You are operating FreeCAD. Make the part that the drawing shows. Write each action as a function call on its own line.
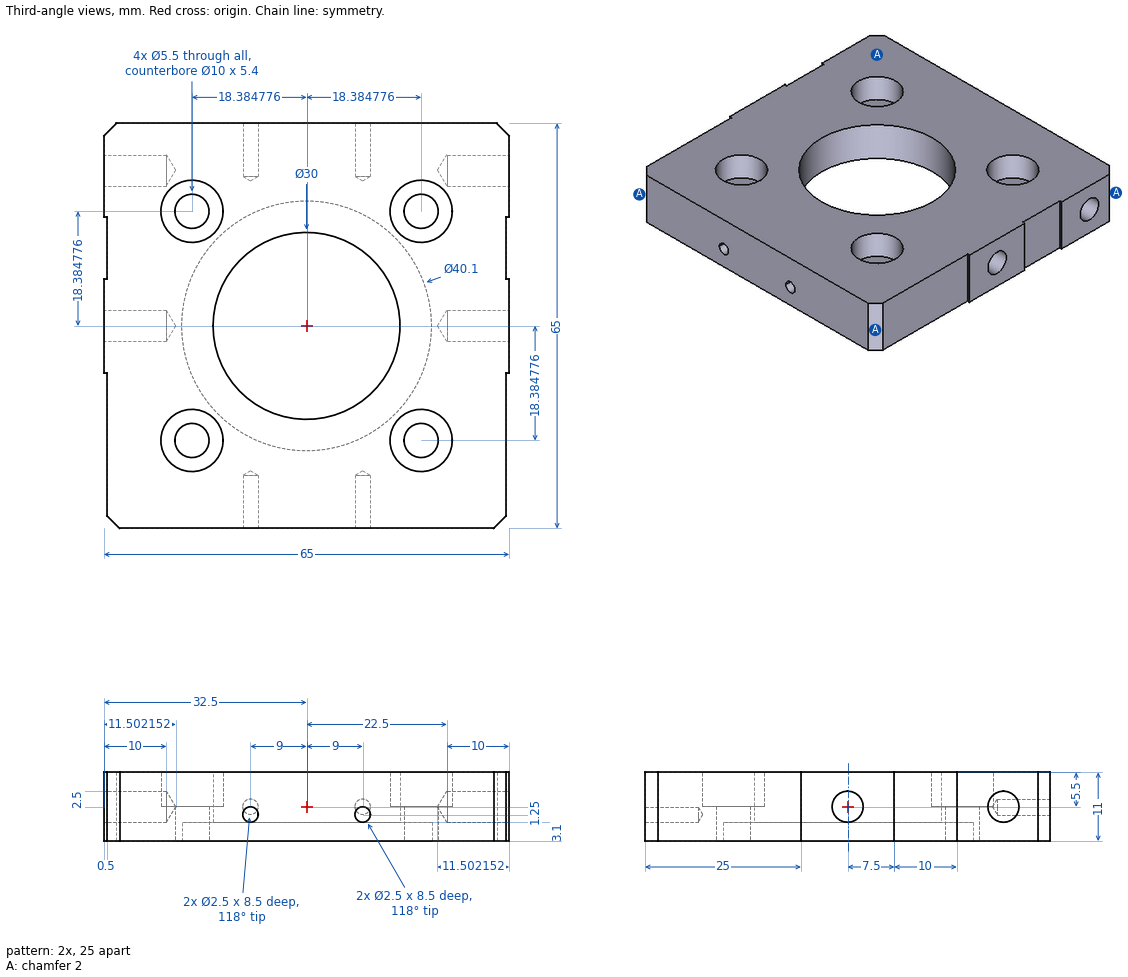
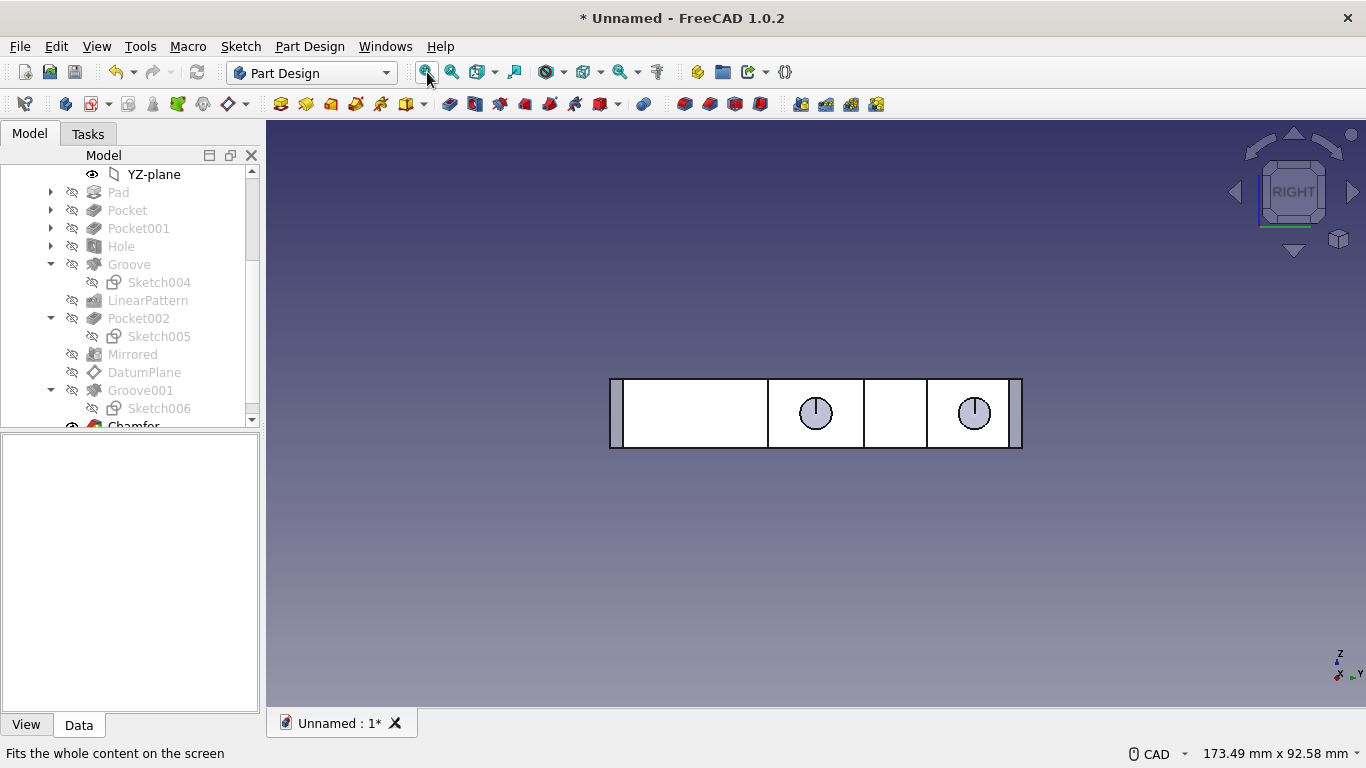
key(4)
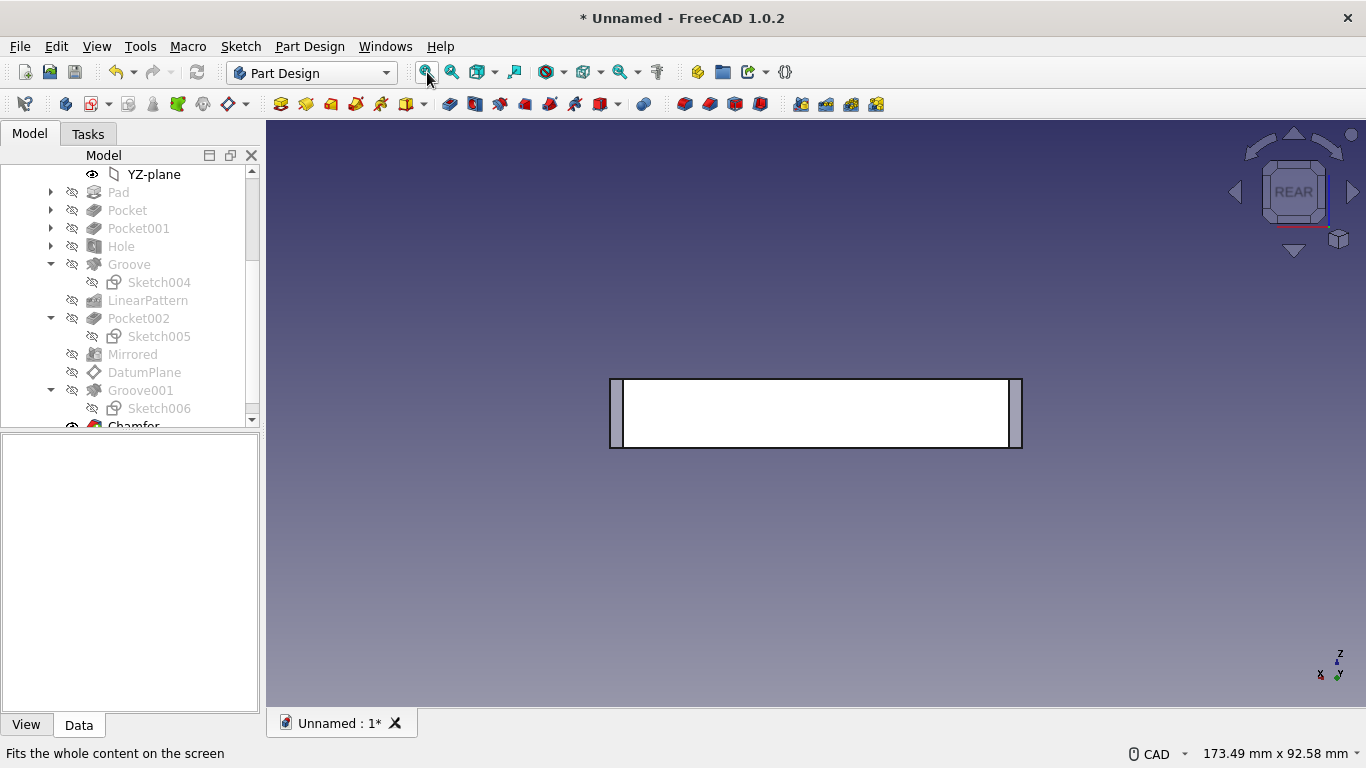
click(427, 72)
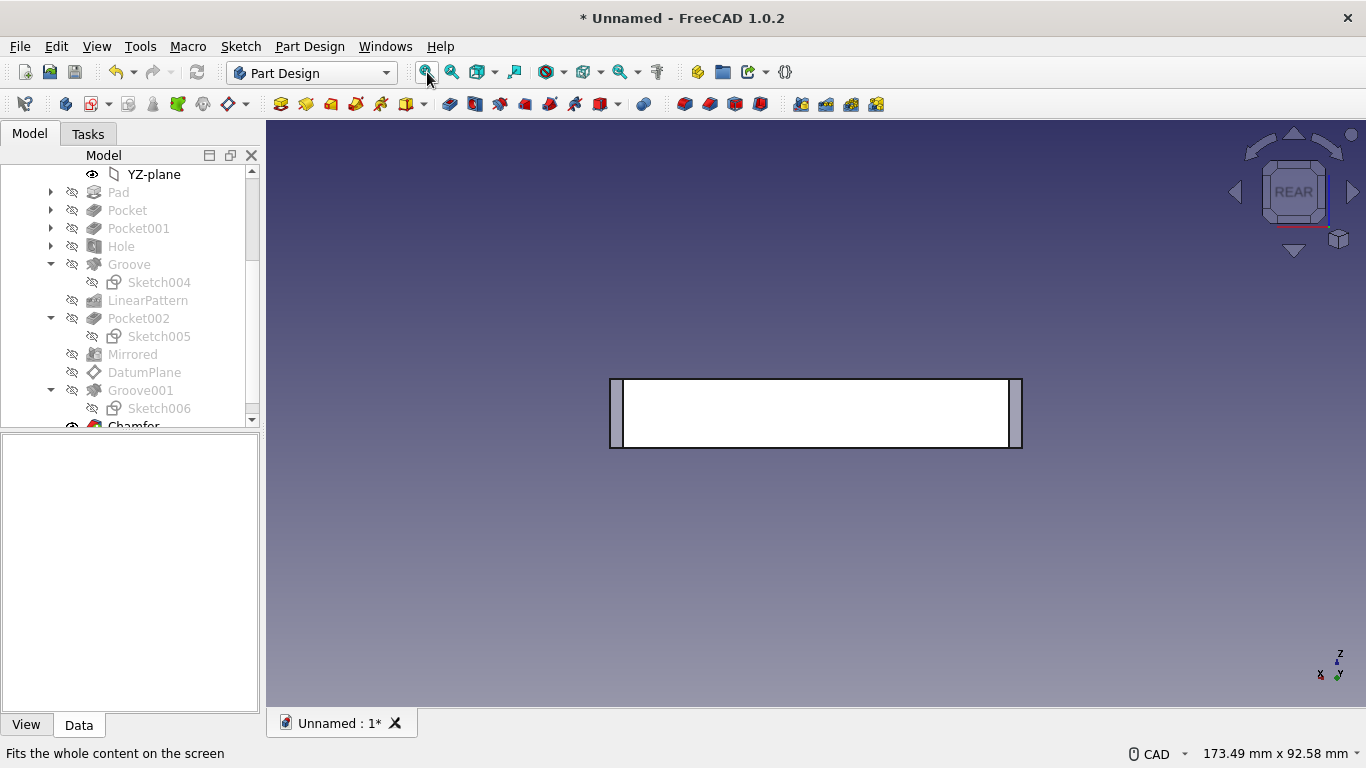
click(705, 413)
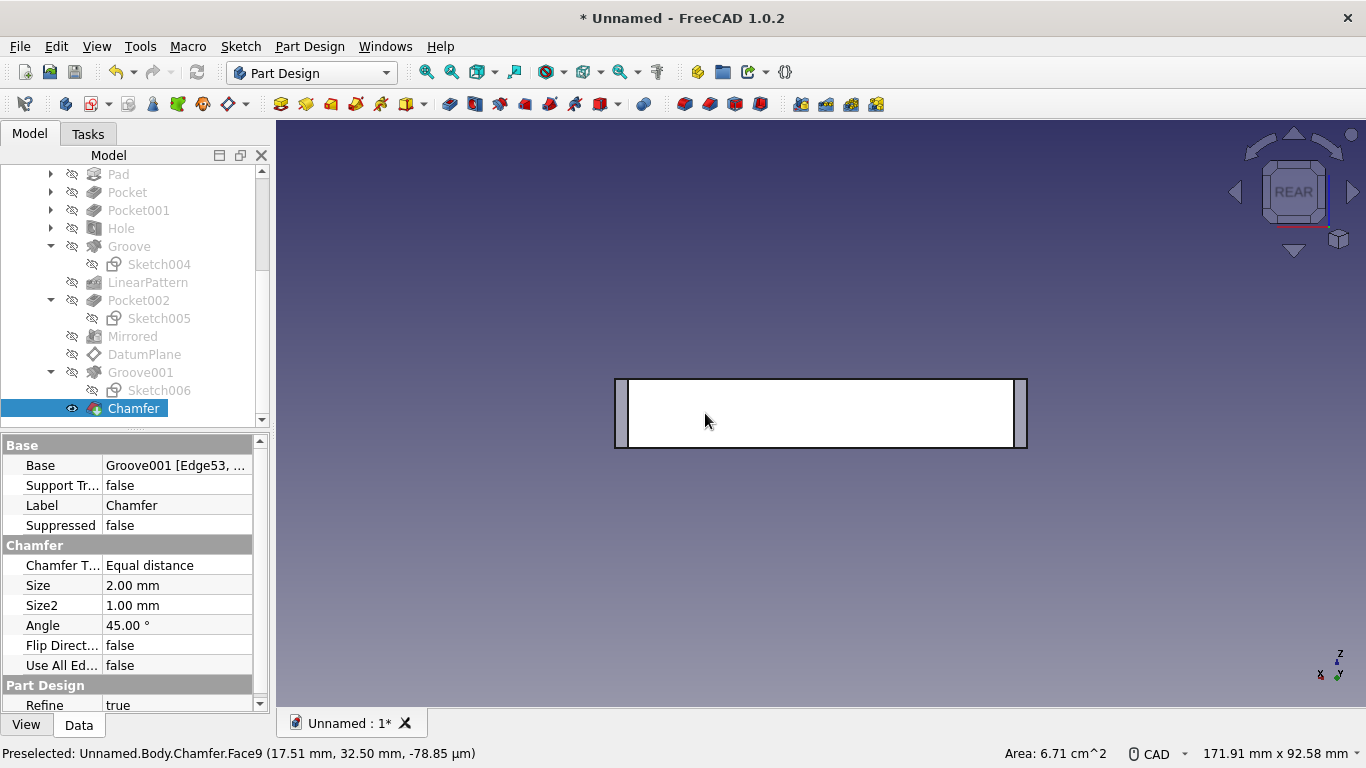
click(90, 104)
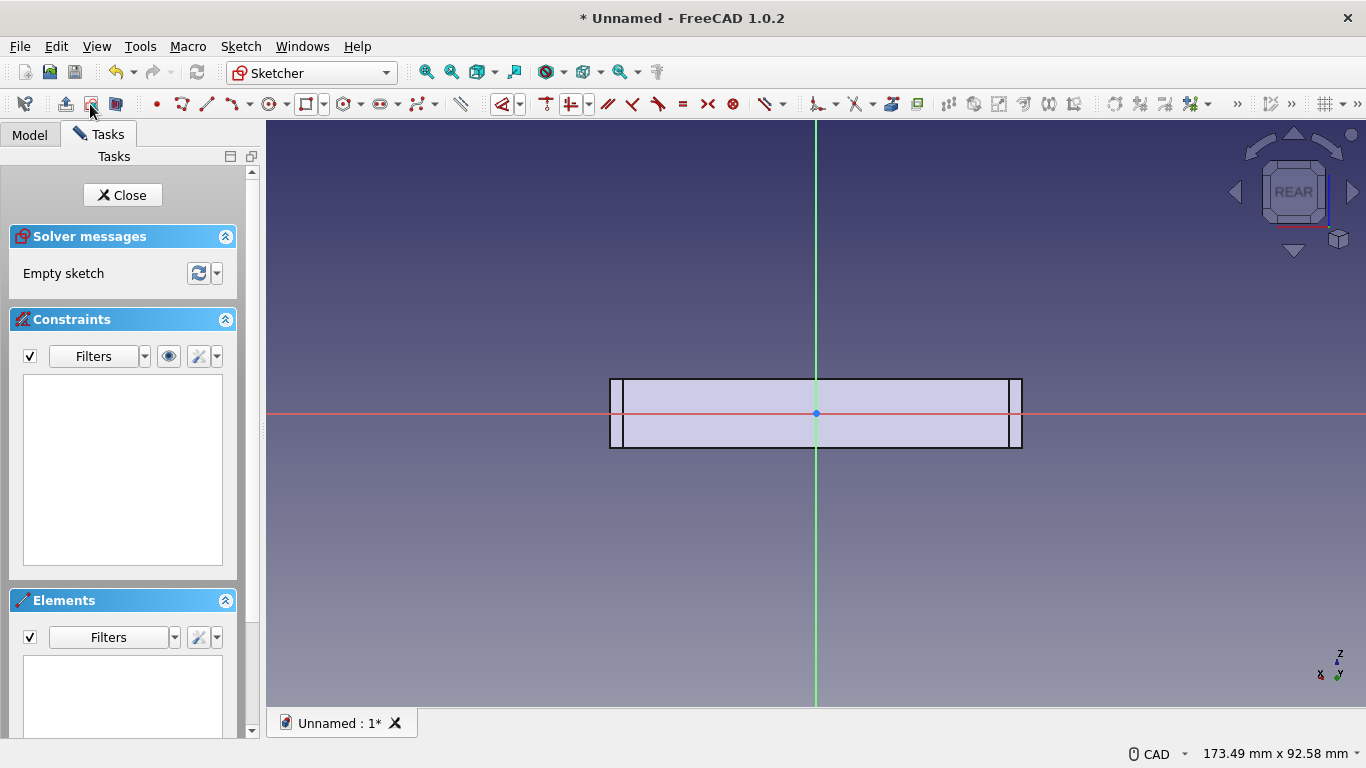
scroll(833, 414, up, 8)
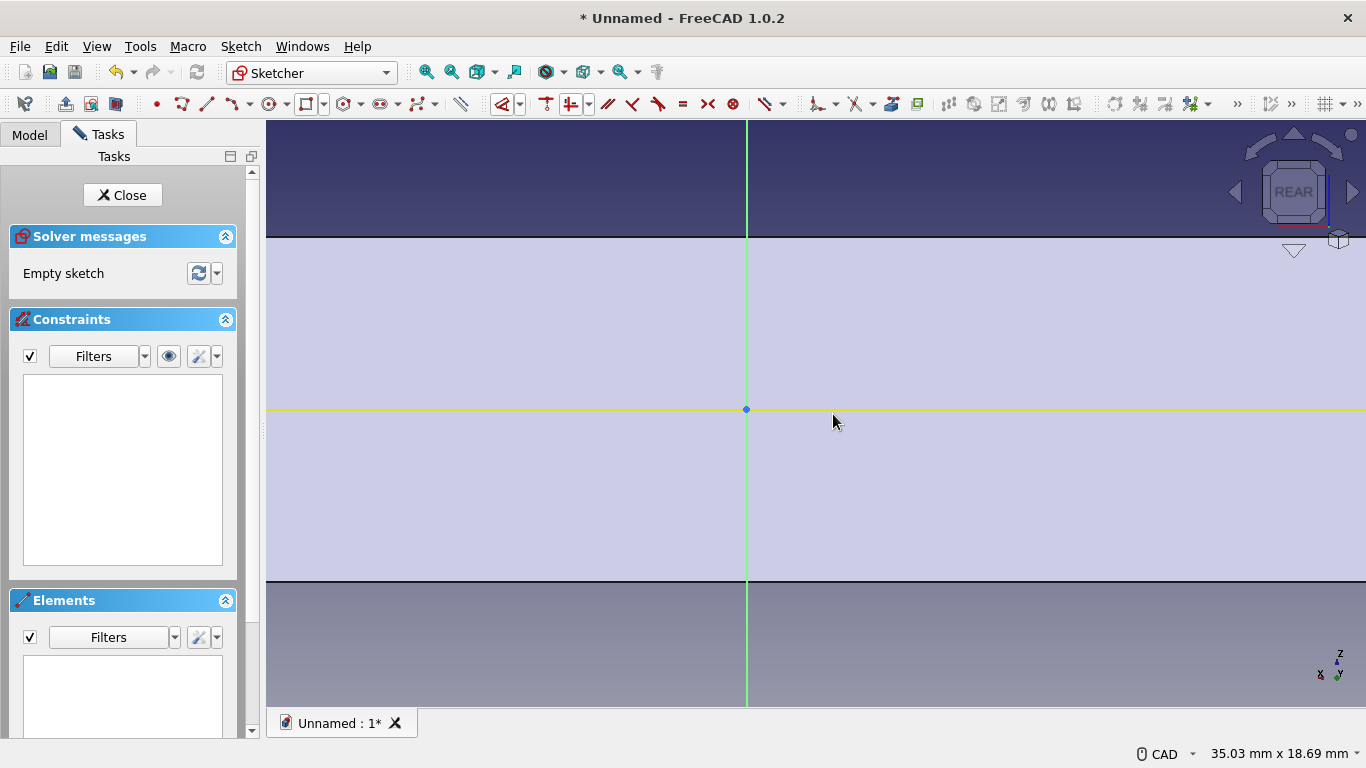
click(268, 104)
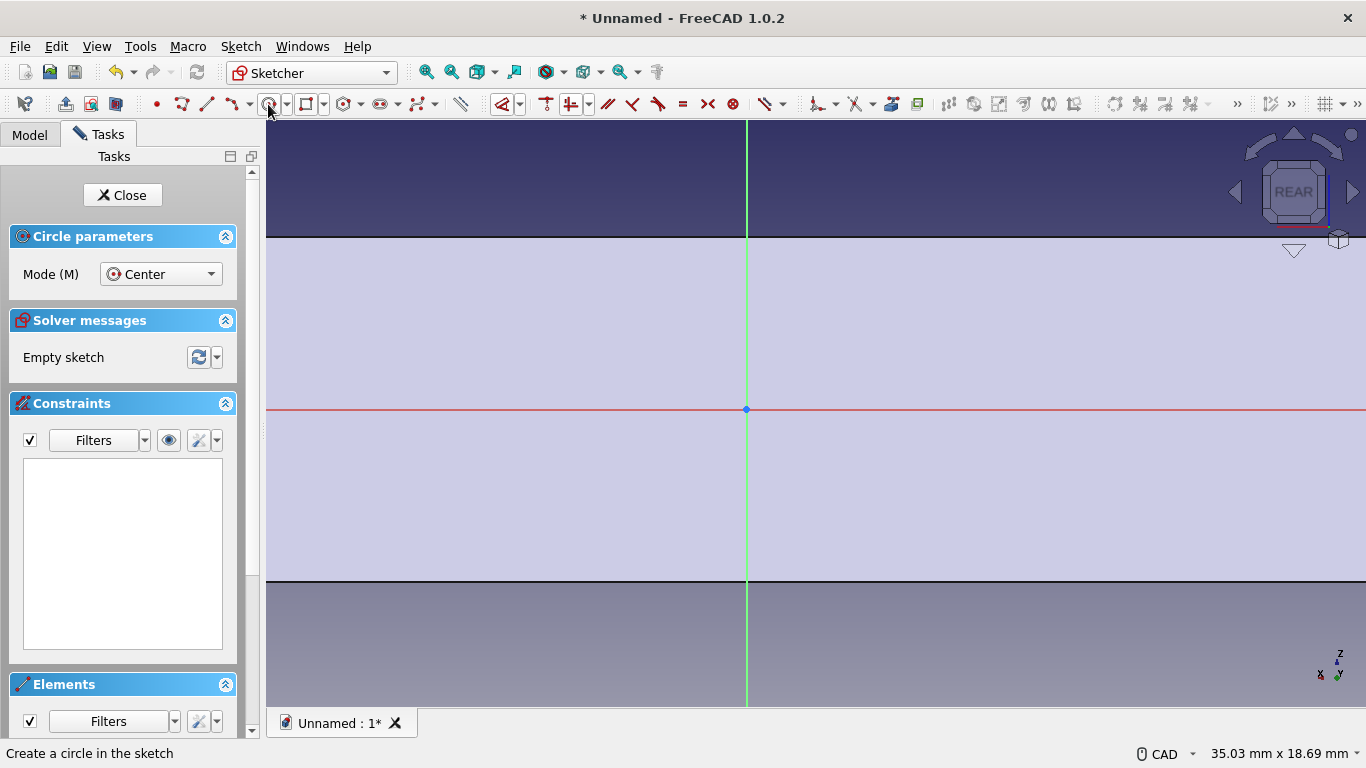
click(1029, 410)
click(1057, 382)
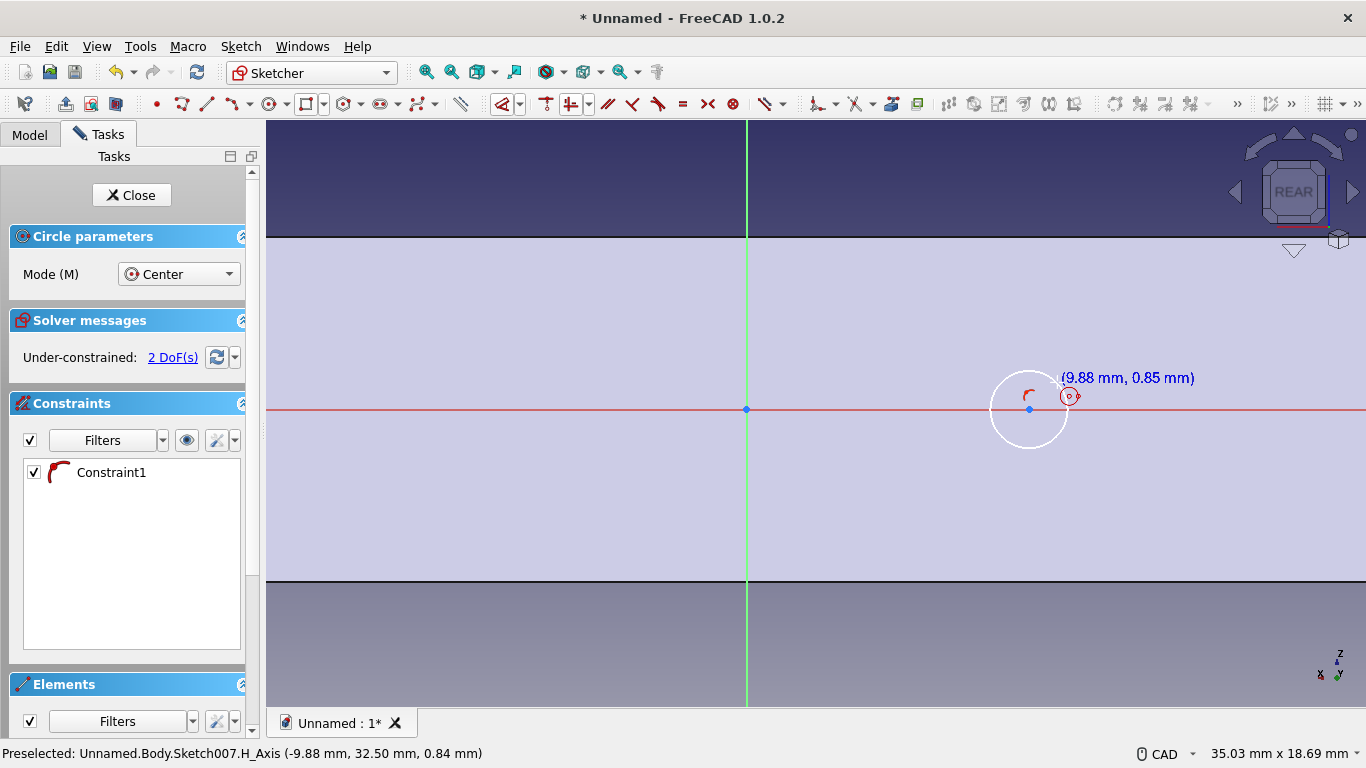
click(464, 410)
click(492, 382)
key(Escape)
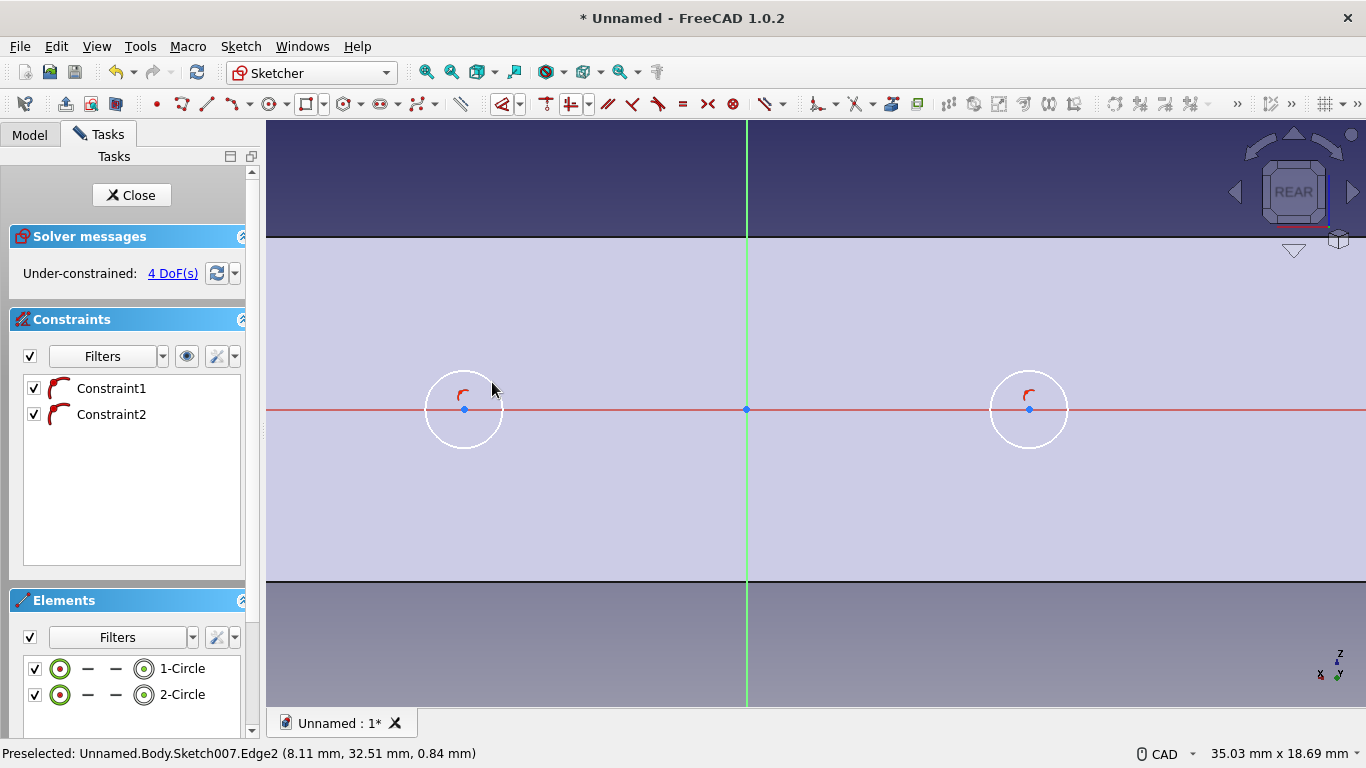
click(1056, 382)